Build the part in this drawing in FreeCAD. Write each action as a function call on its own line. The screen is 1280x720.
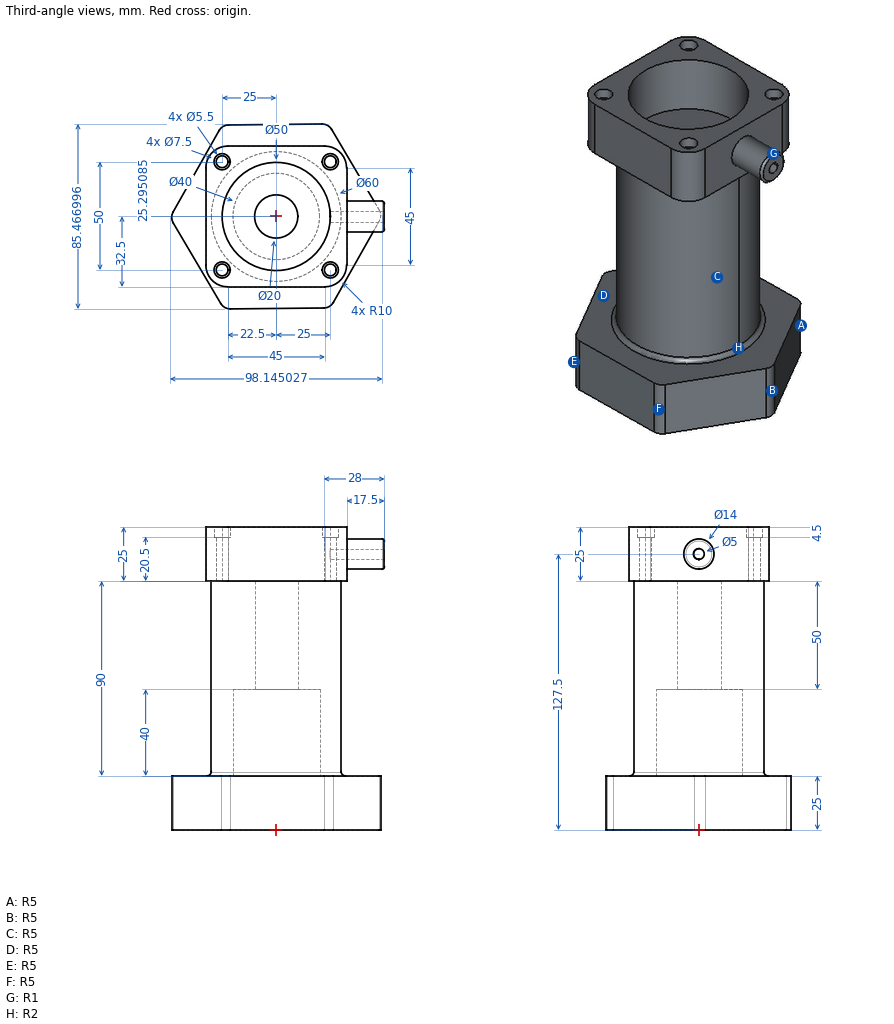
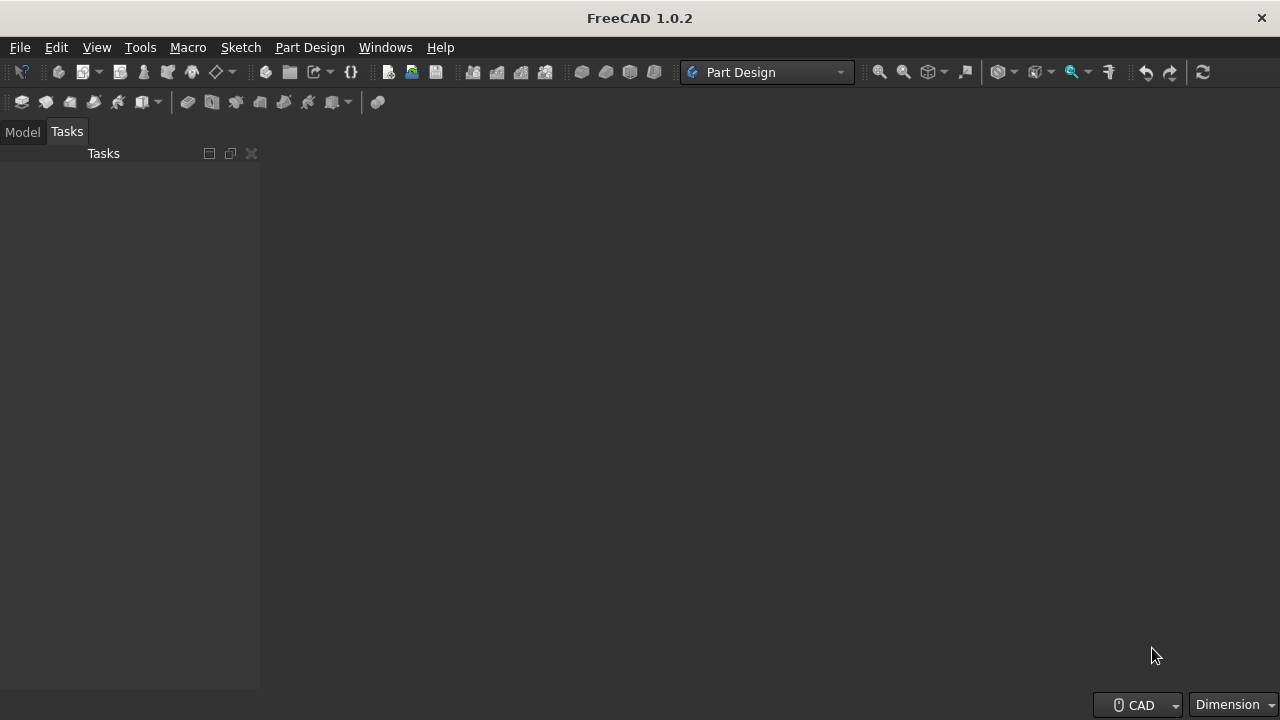
click(388, 72)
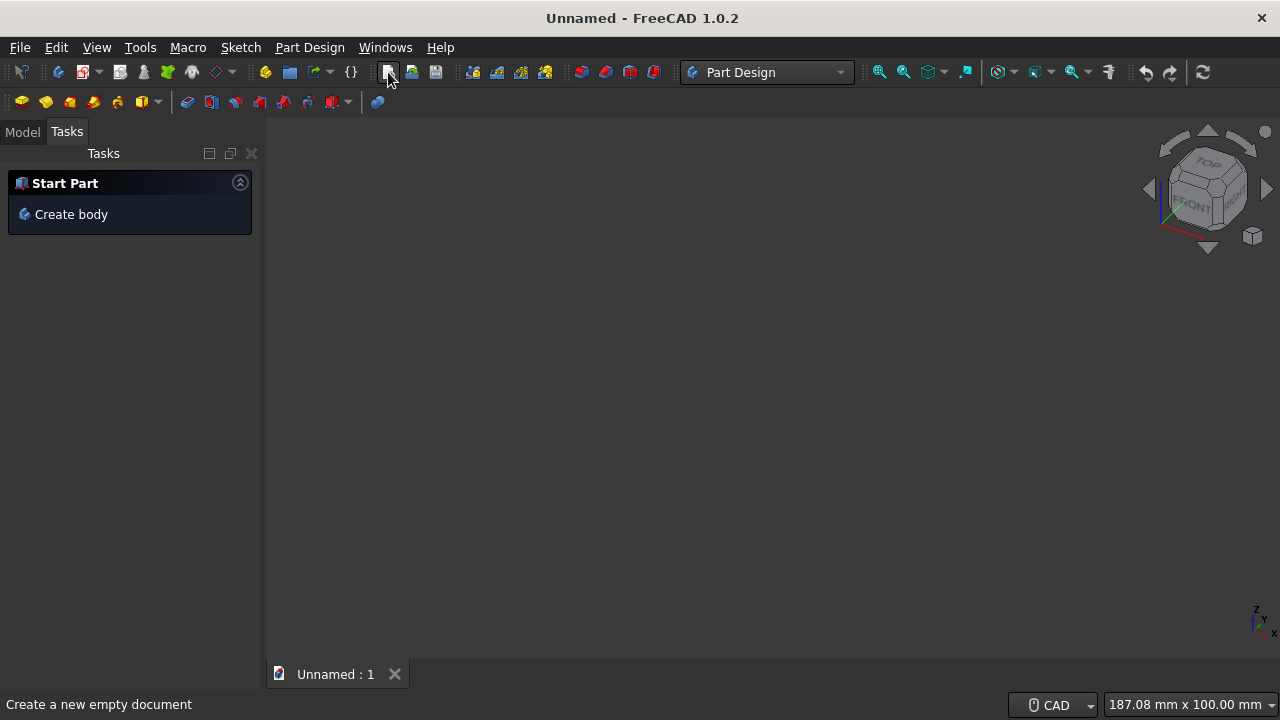
click(84, 72)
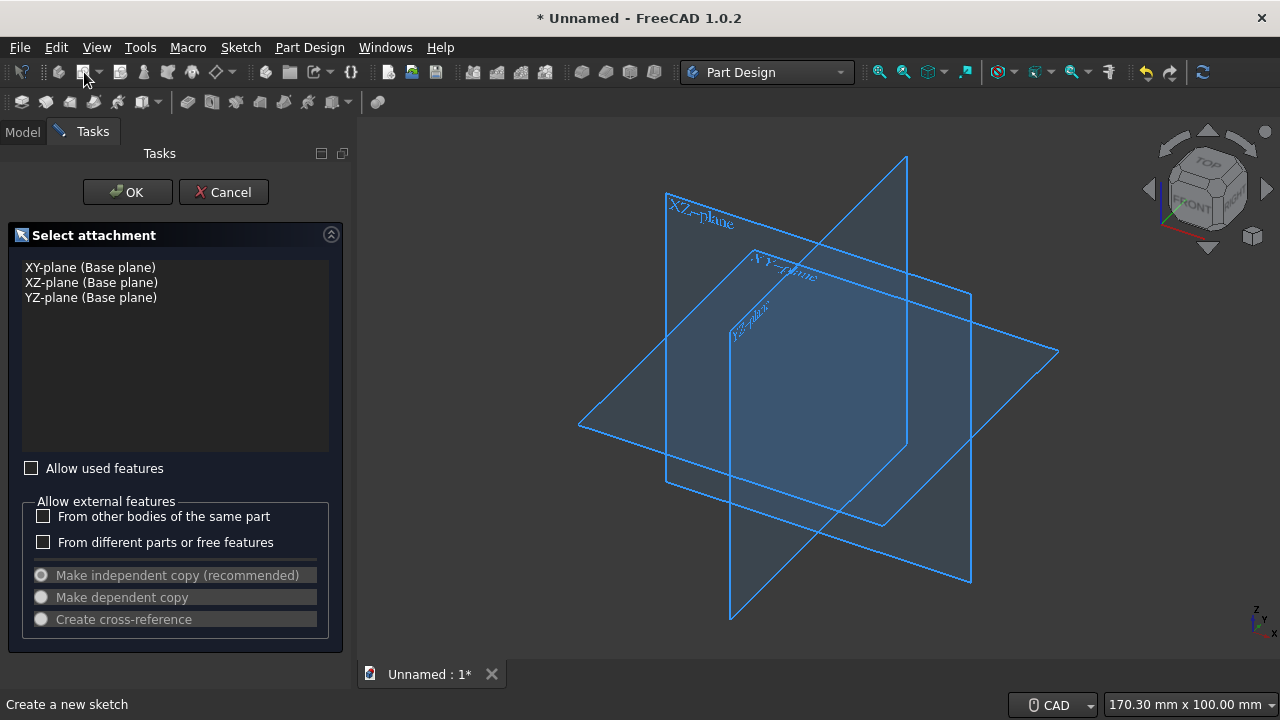
click(82, 268)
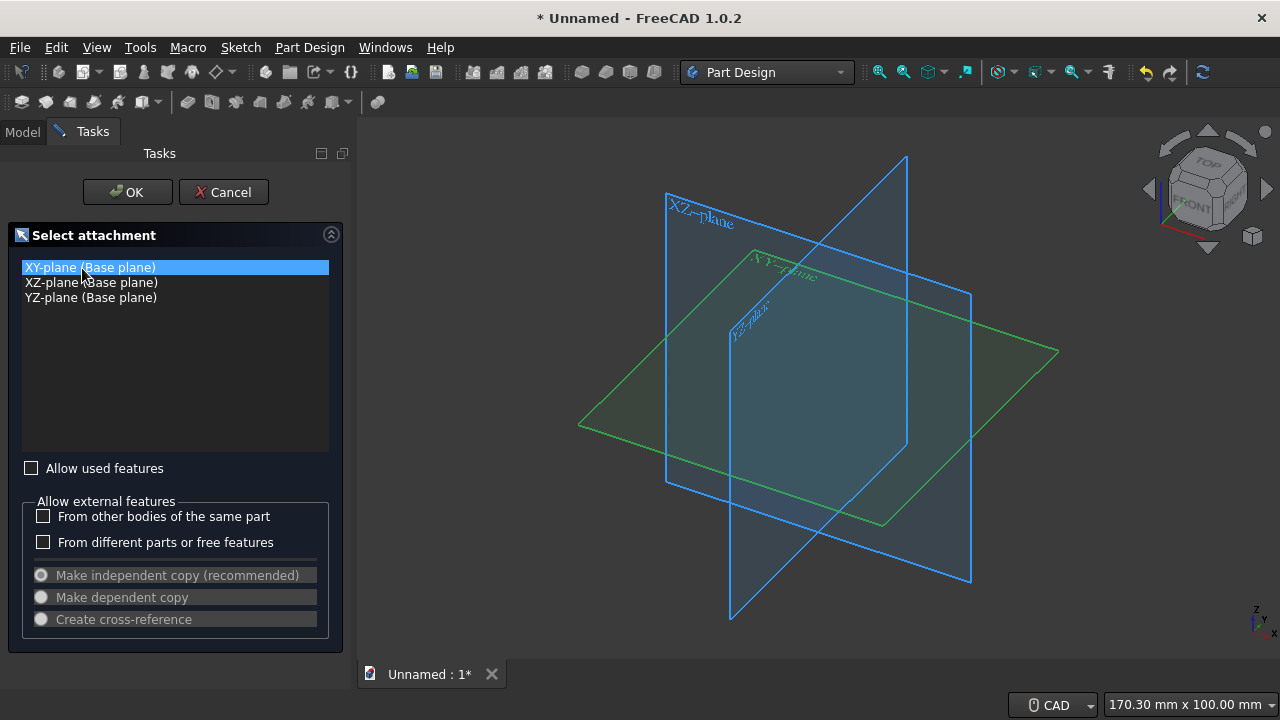
click(128, 192)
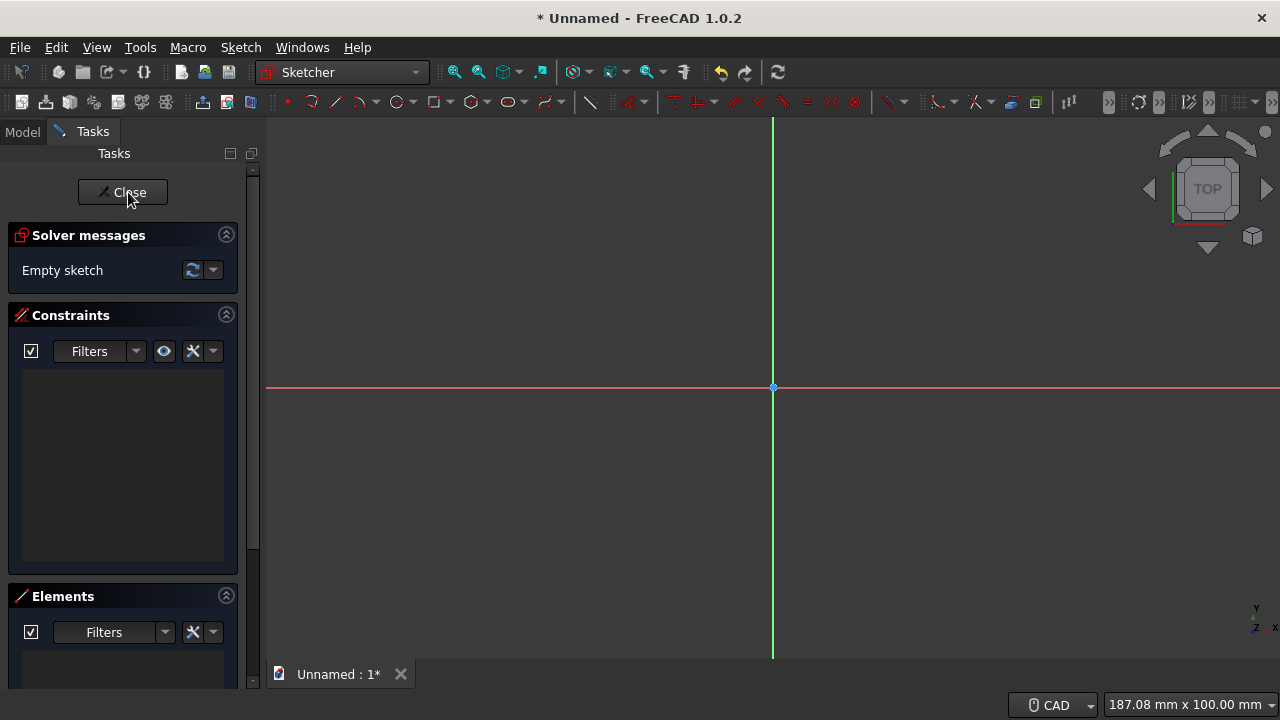
scroll(565, 388, down, 2)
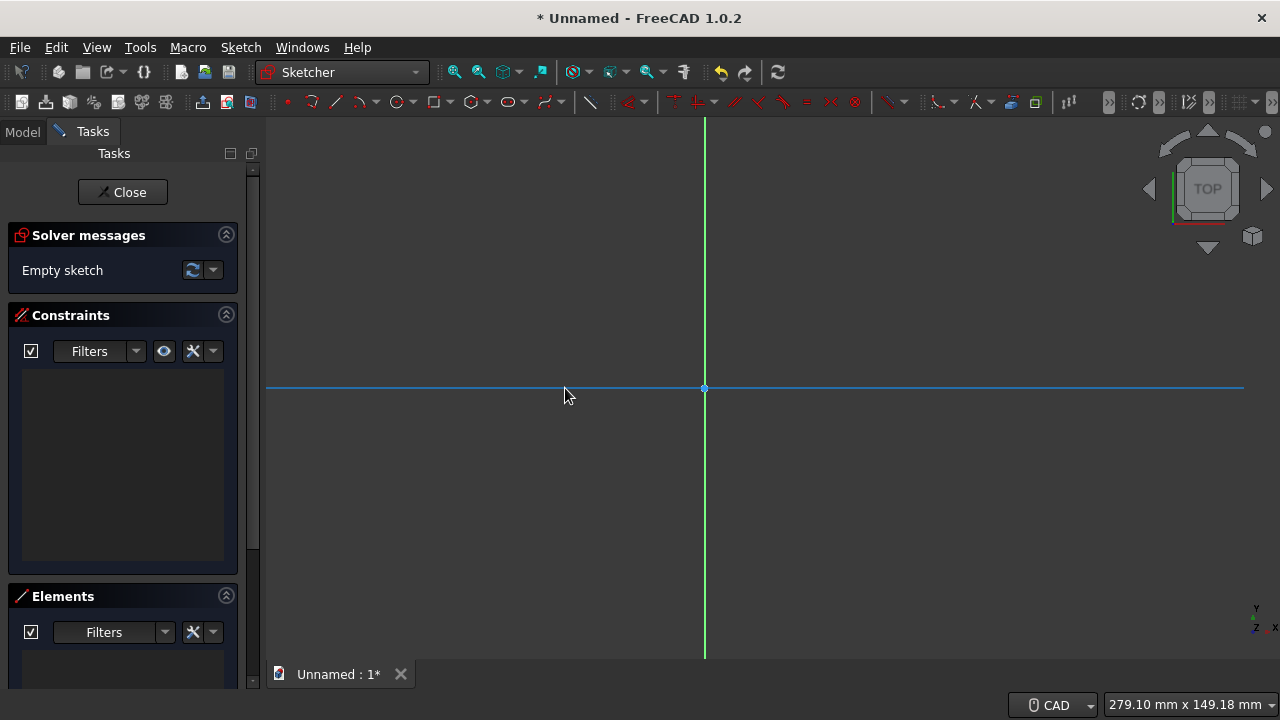
click(472, 102)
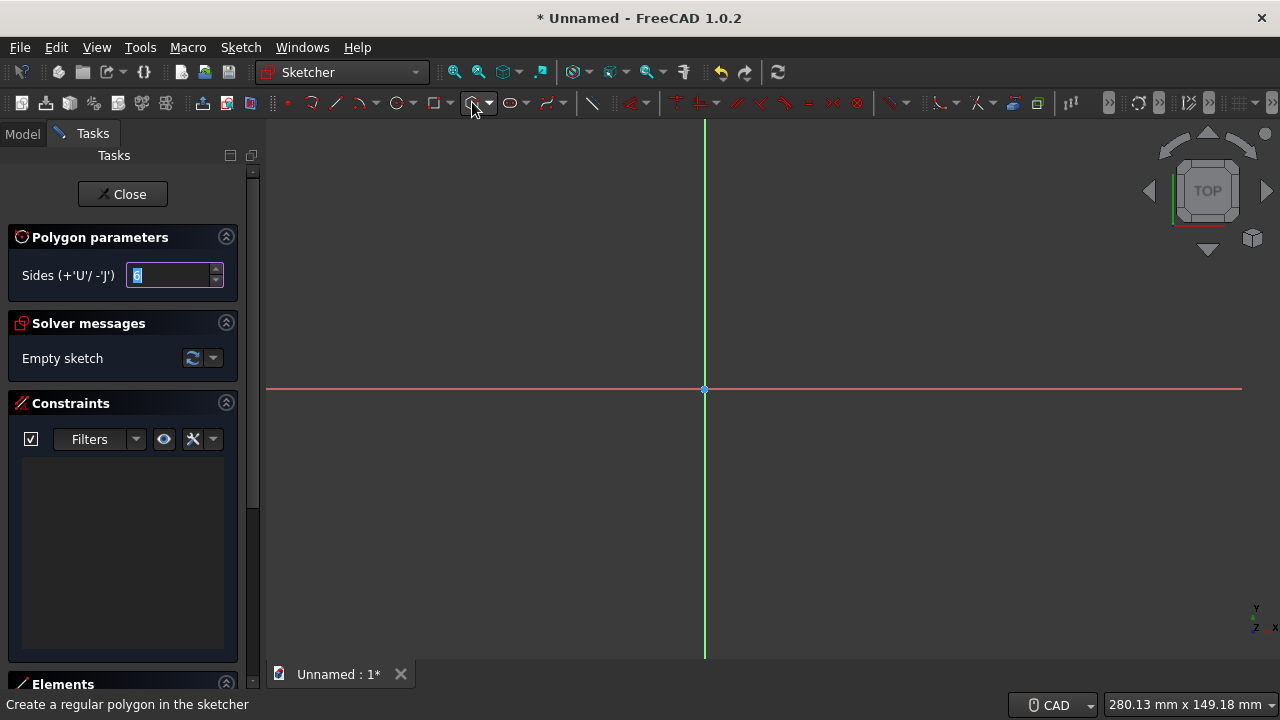
click(705, 389)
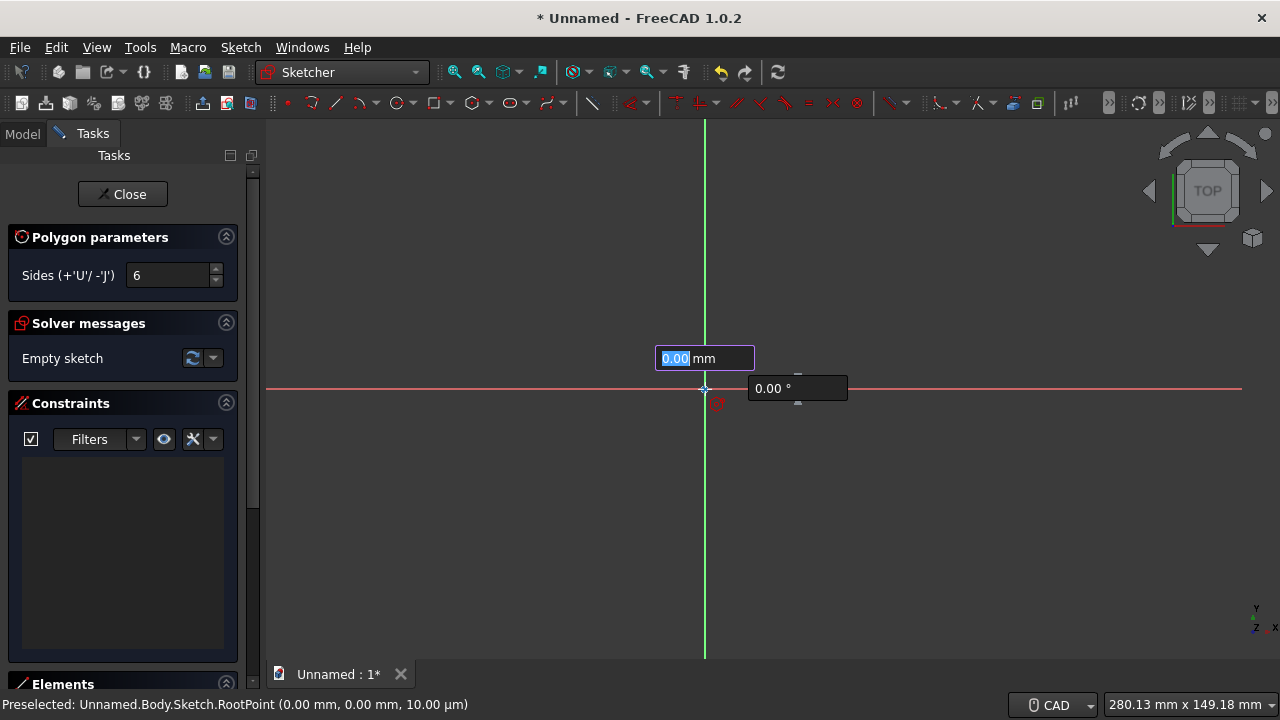
click(614, 236)
right_click(614, 236)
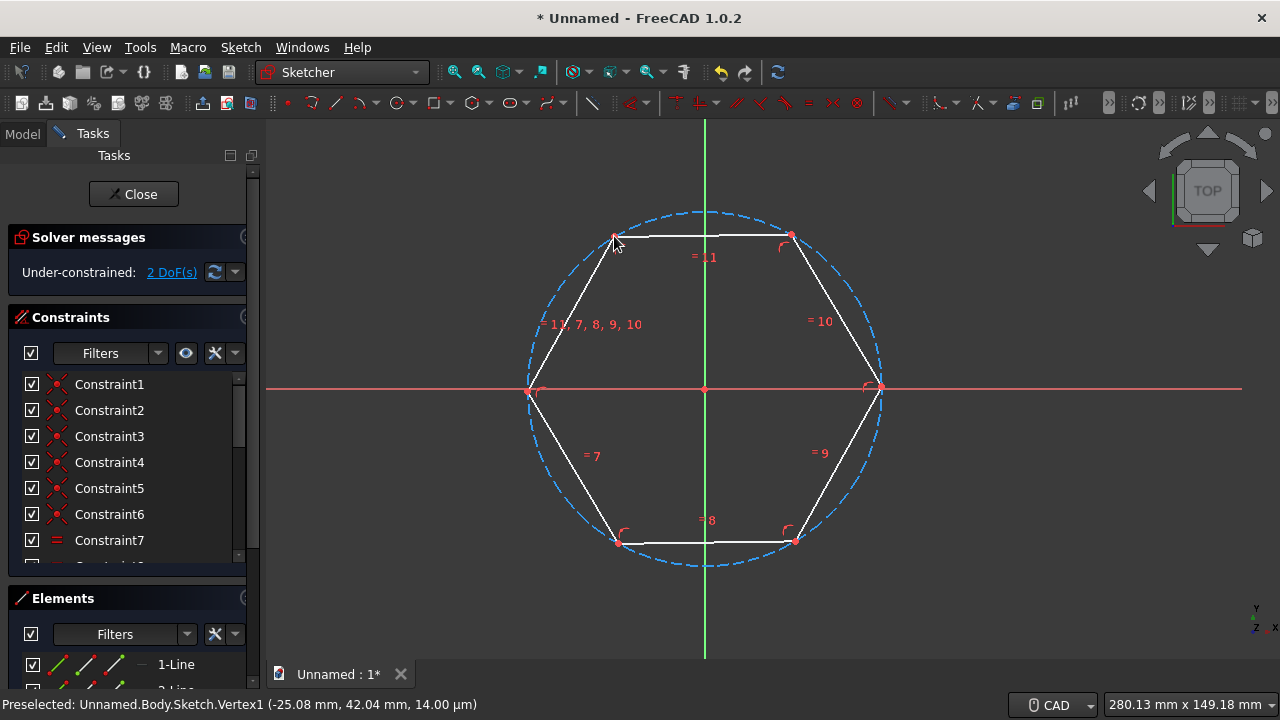
click(630, 104)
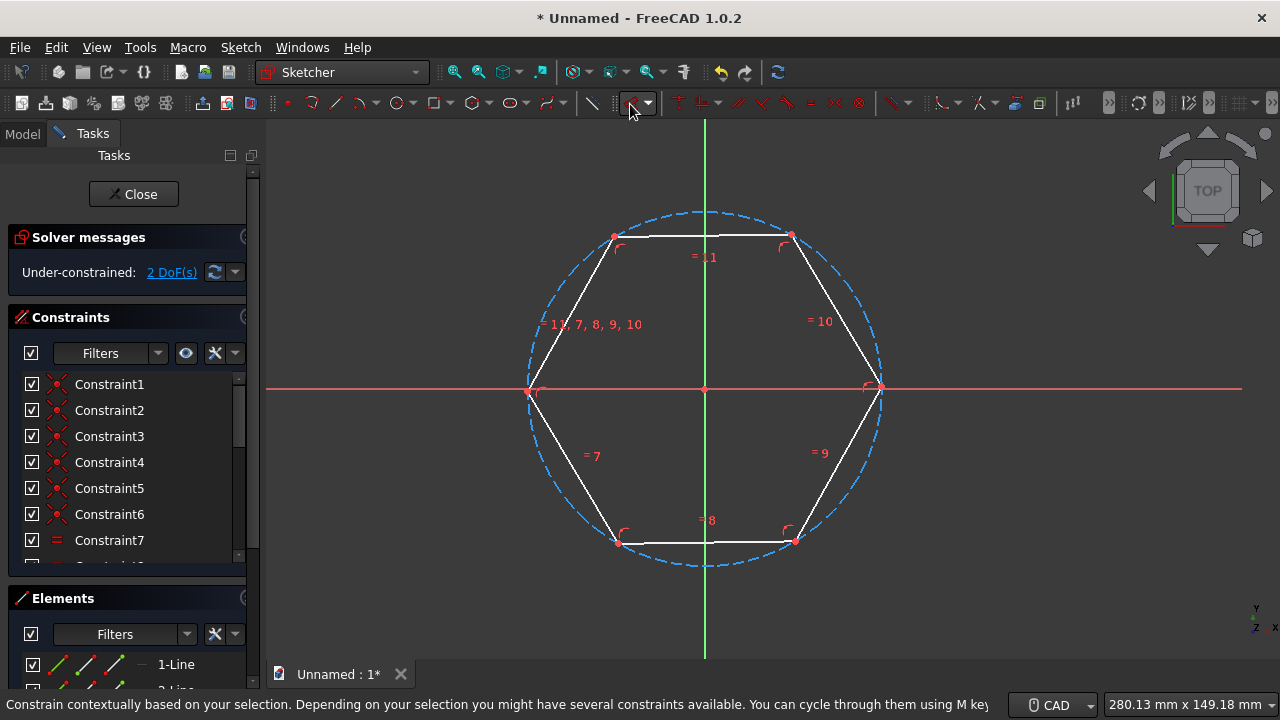
click(618, 544)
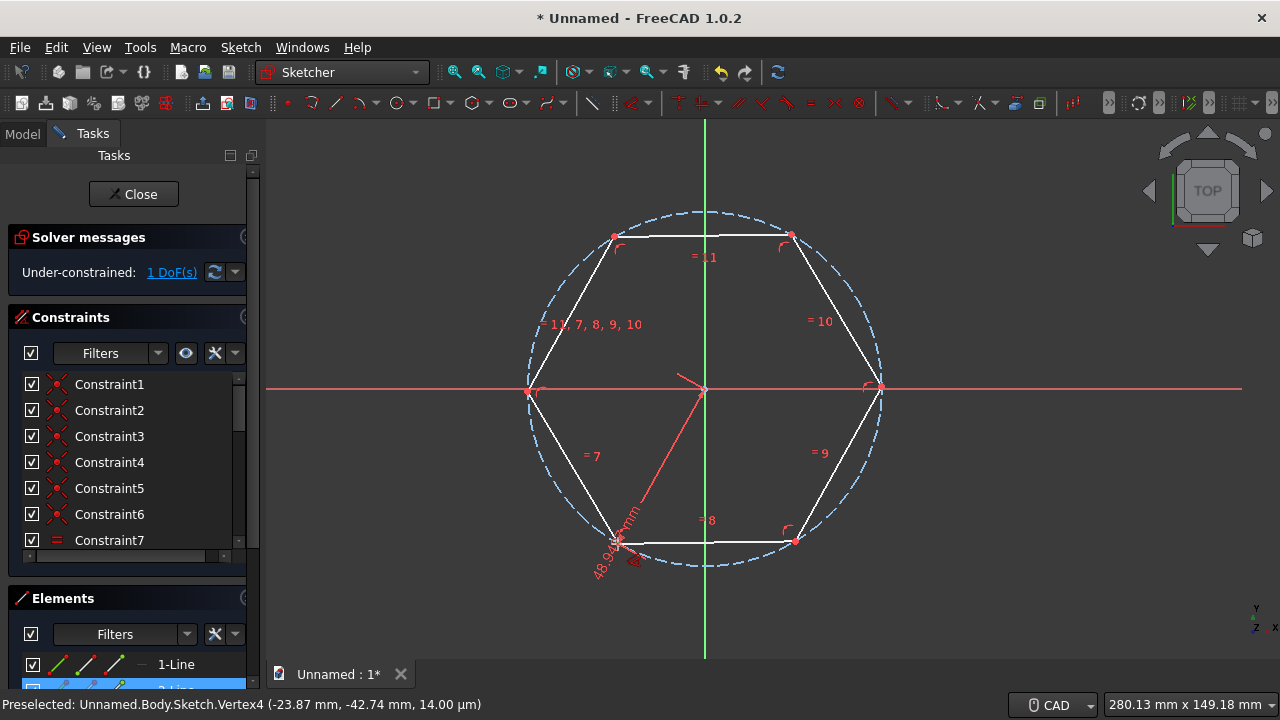
click(791, 234)
click(825, 318)